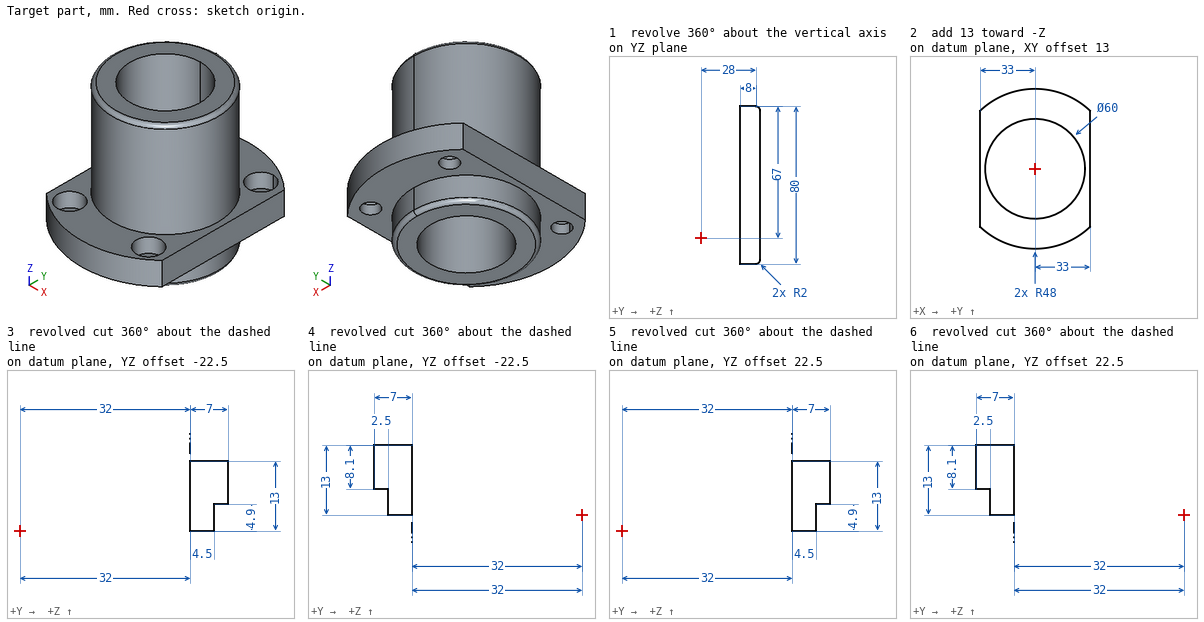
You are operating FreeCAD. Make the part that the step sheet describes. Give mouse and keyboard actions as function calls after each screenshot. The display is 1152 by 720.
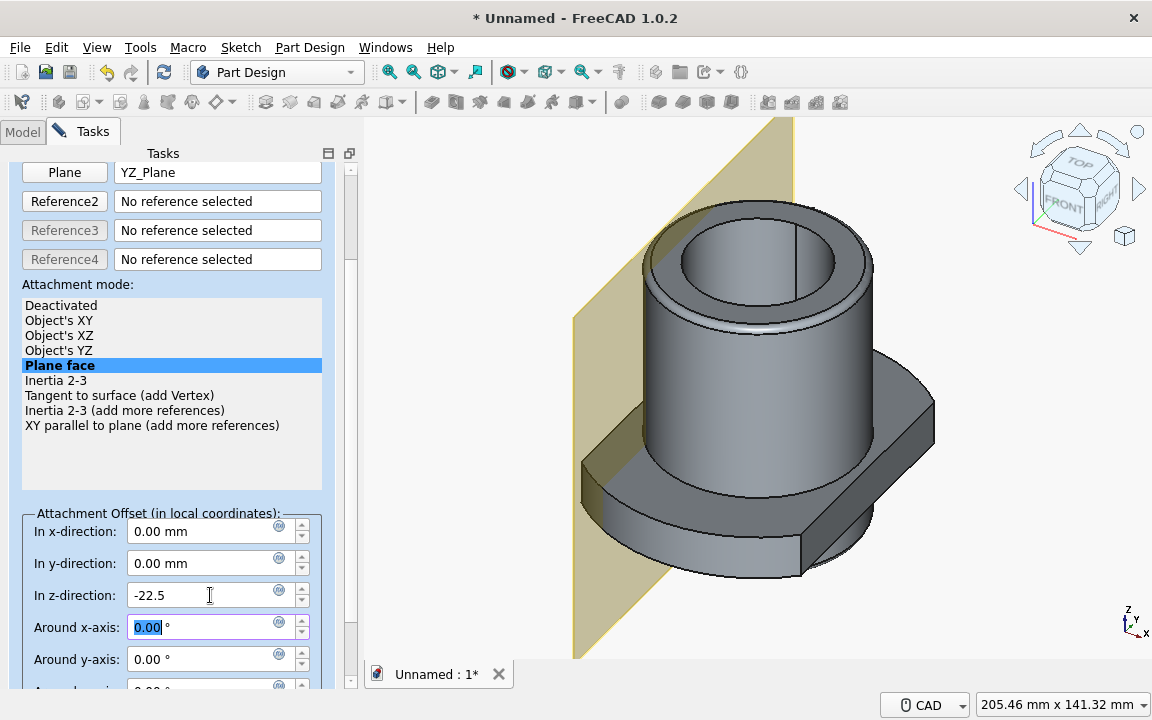
scroll(351, 426, up, 3)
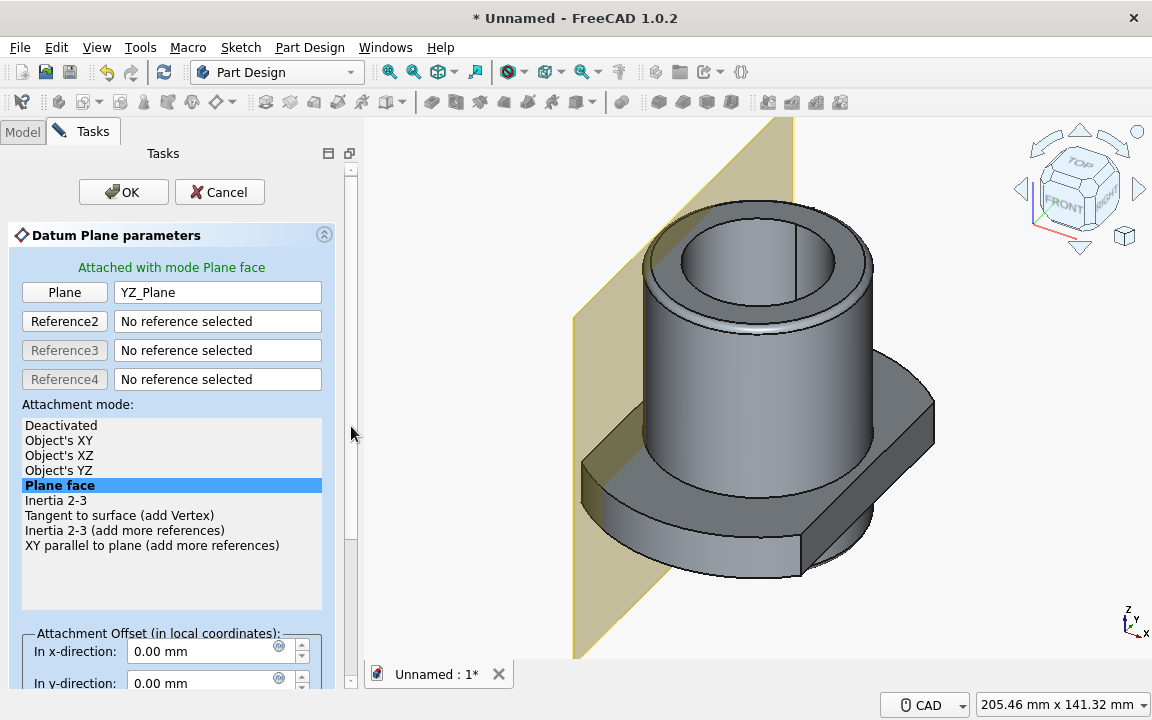
click(124, 192)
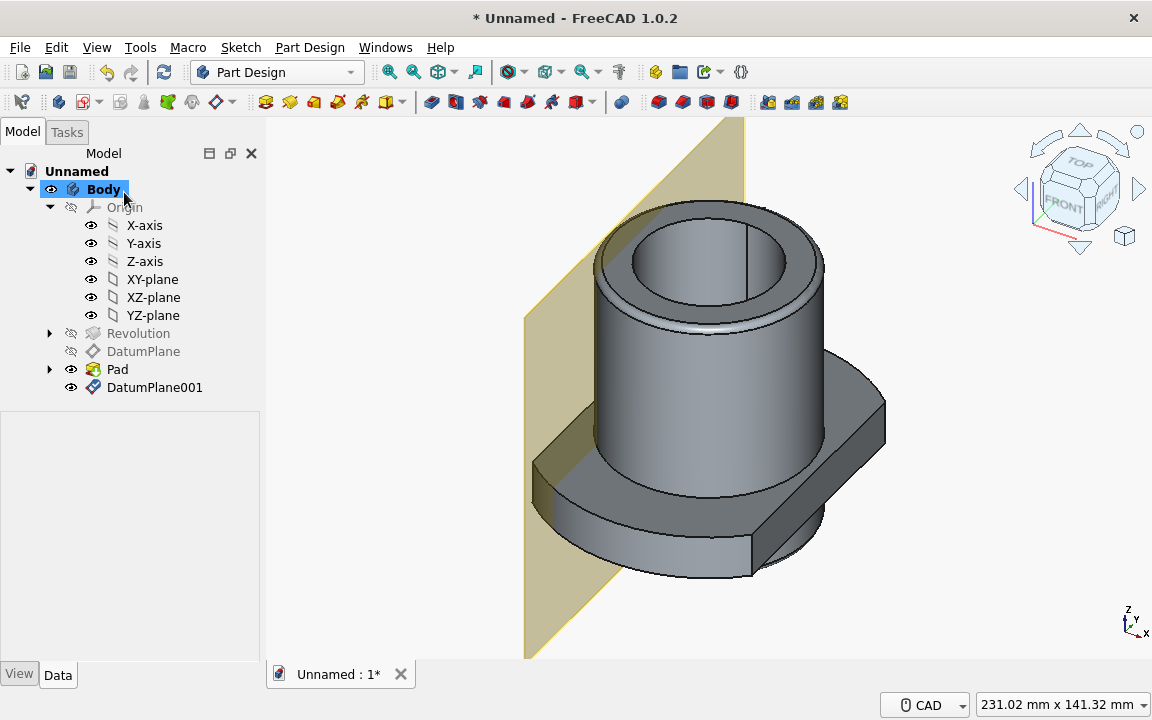
click(116, 387)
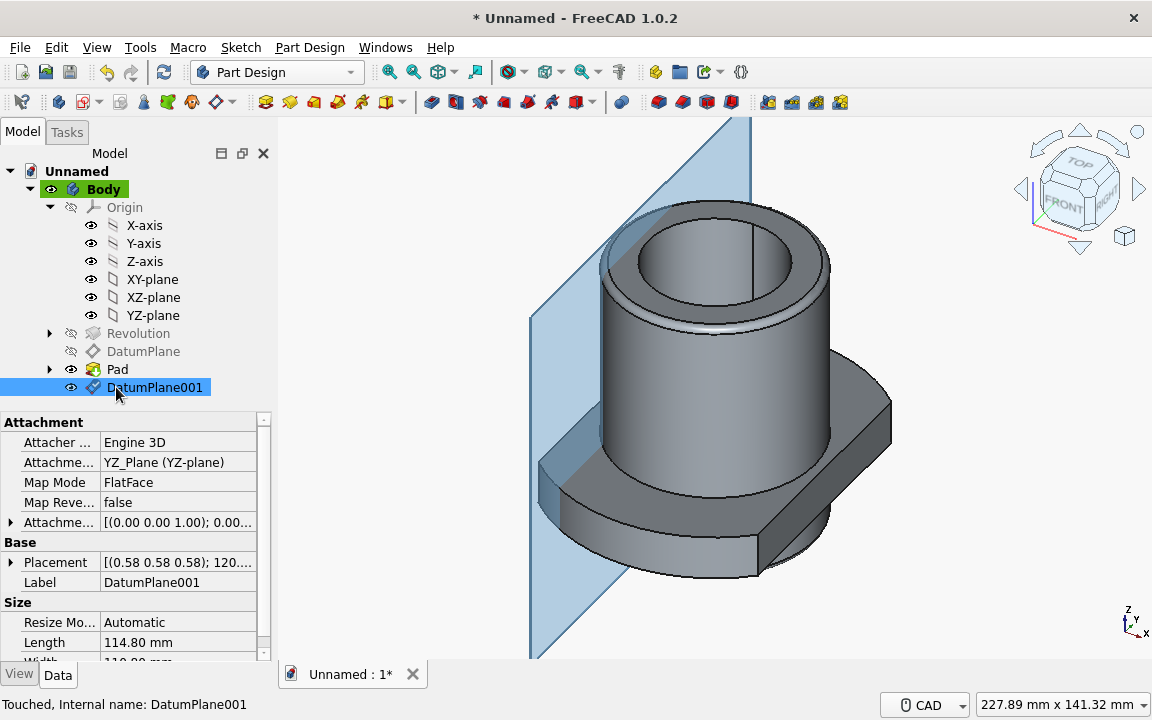
click(84, 102)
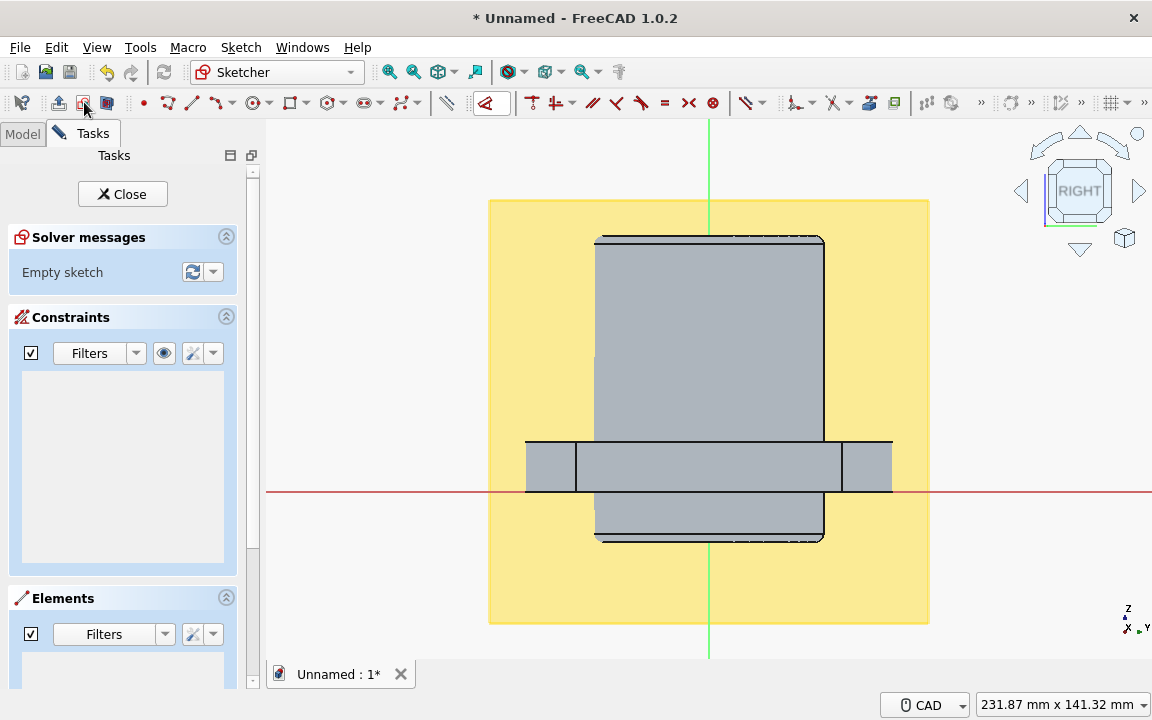
click(108, 104)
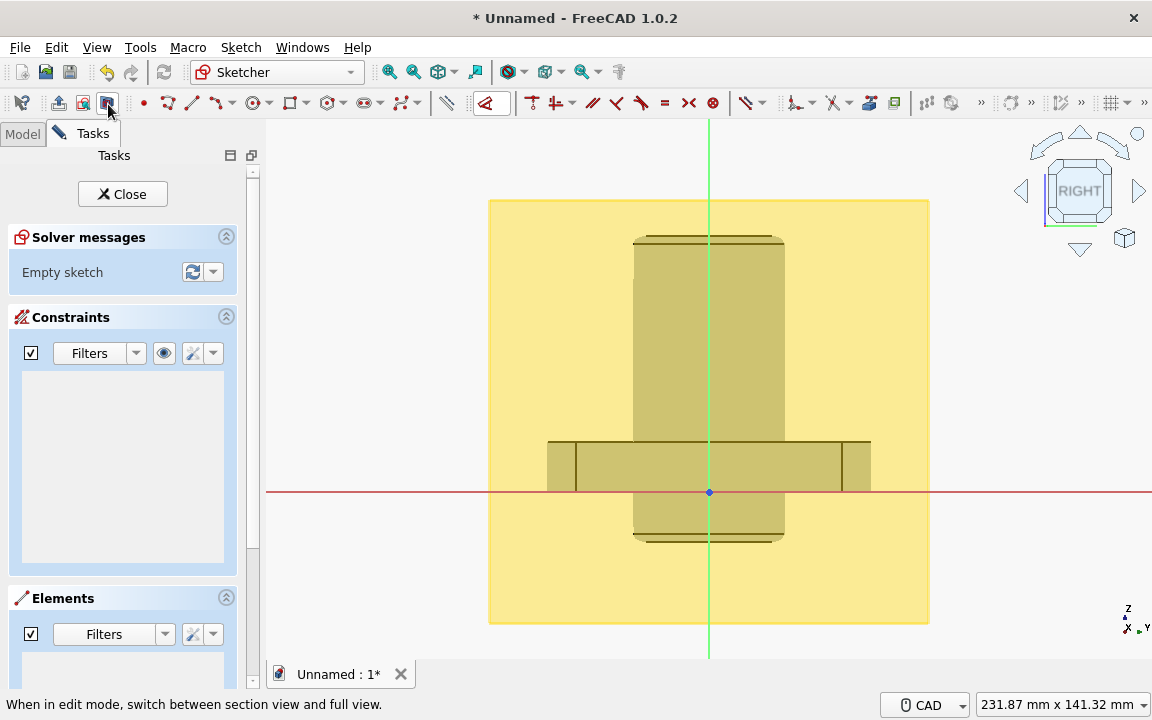
scroll(845, 487, up, 6)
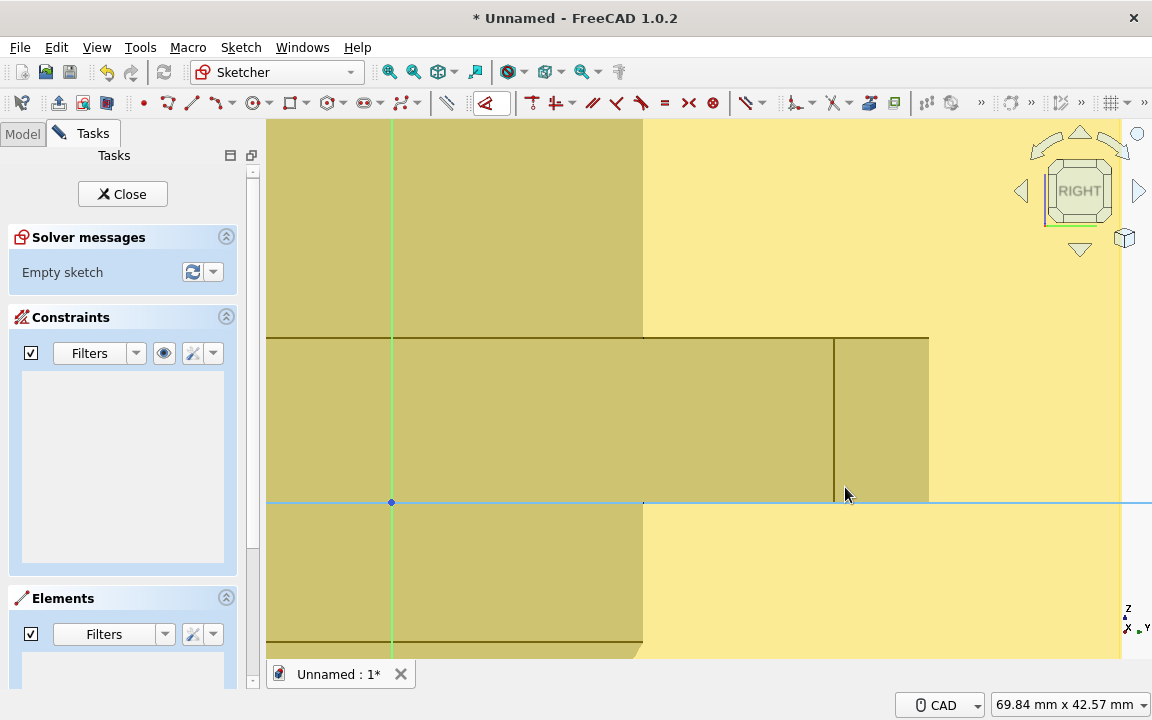
click(168, 104)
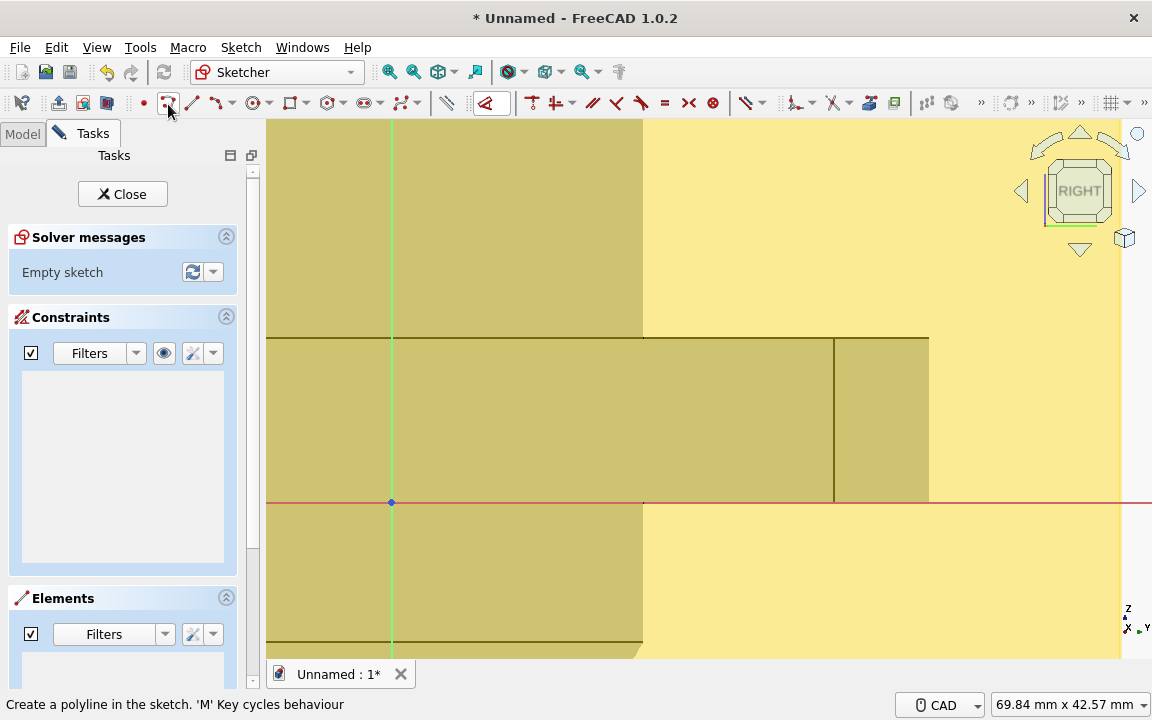
click(798, 503)
click(855, 494)
click(855, 440)
click(887, 440)
click(887, 338)
click(798, 338)
click(798, 503)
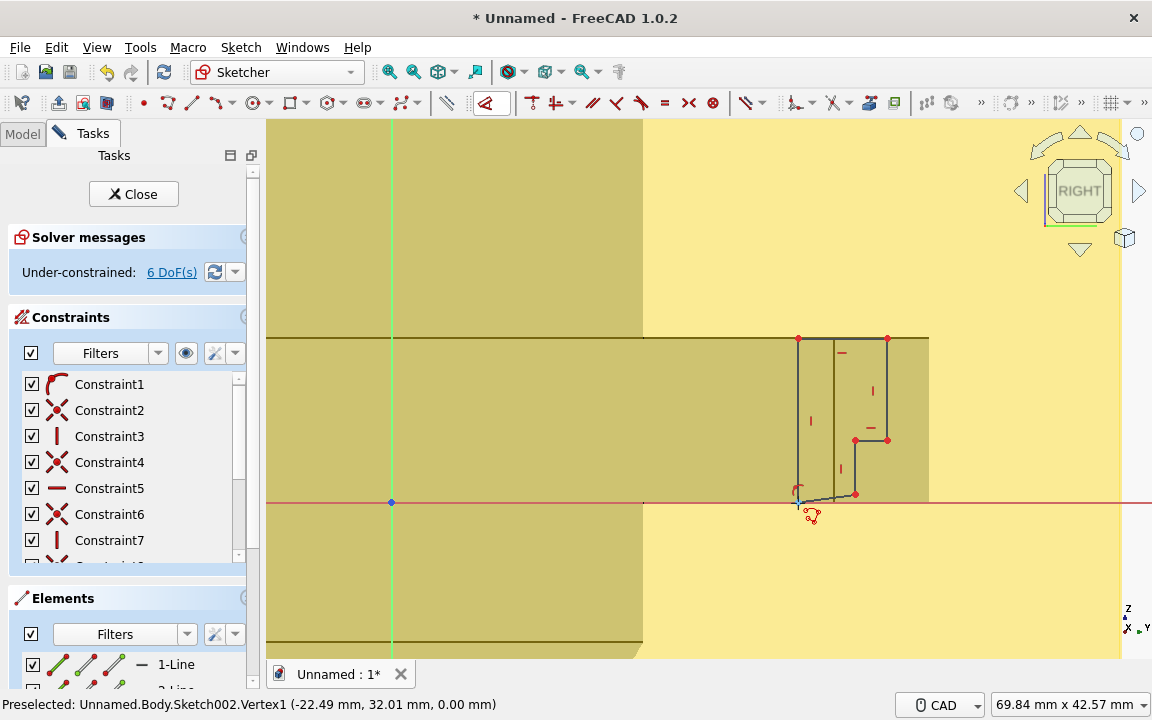
click(192, 104)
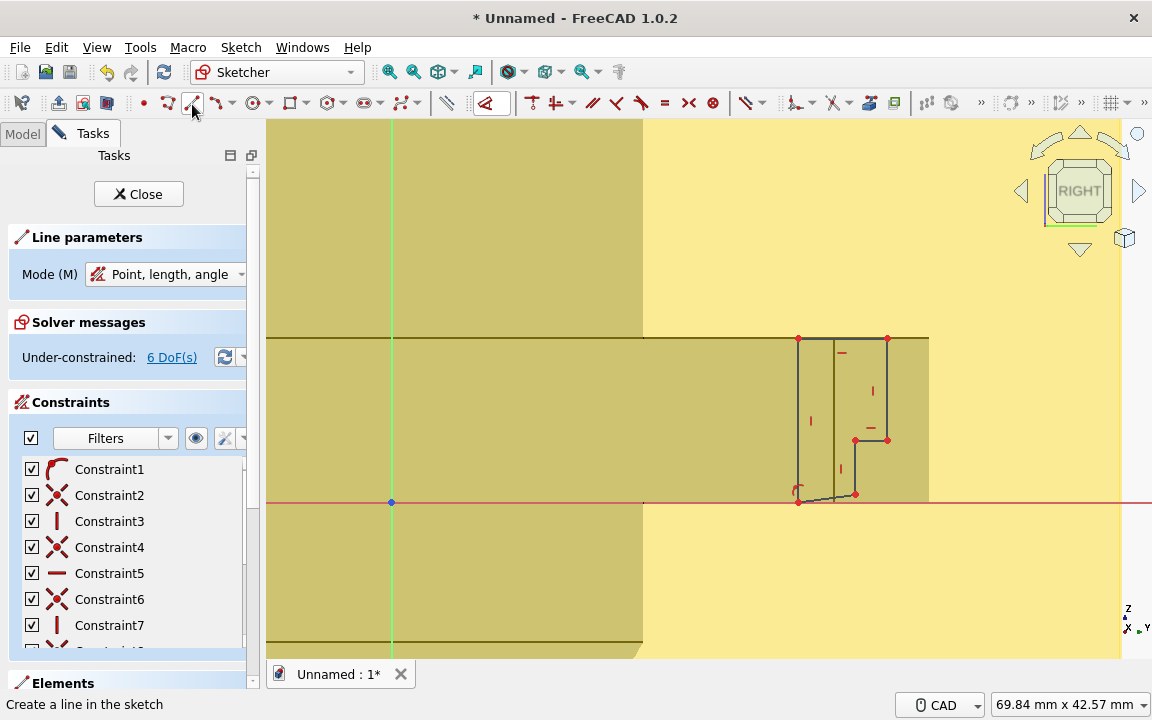
click(798, 321)
click(798, 272)
key(Escape)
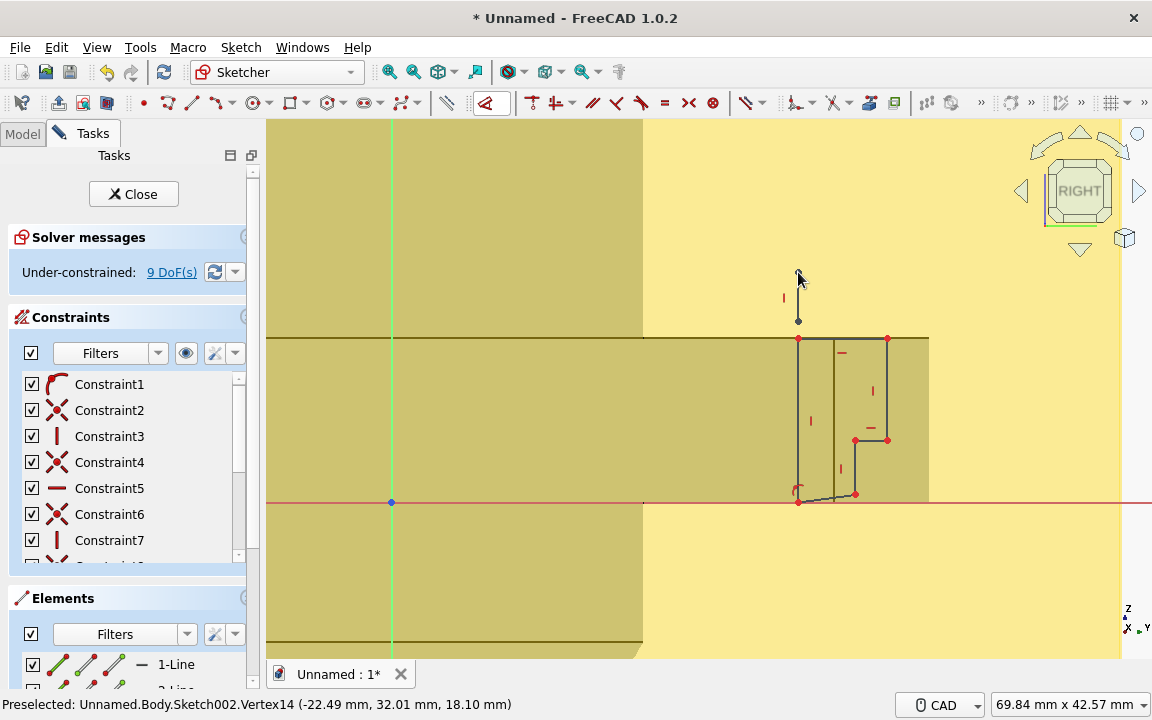
click(798, 307)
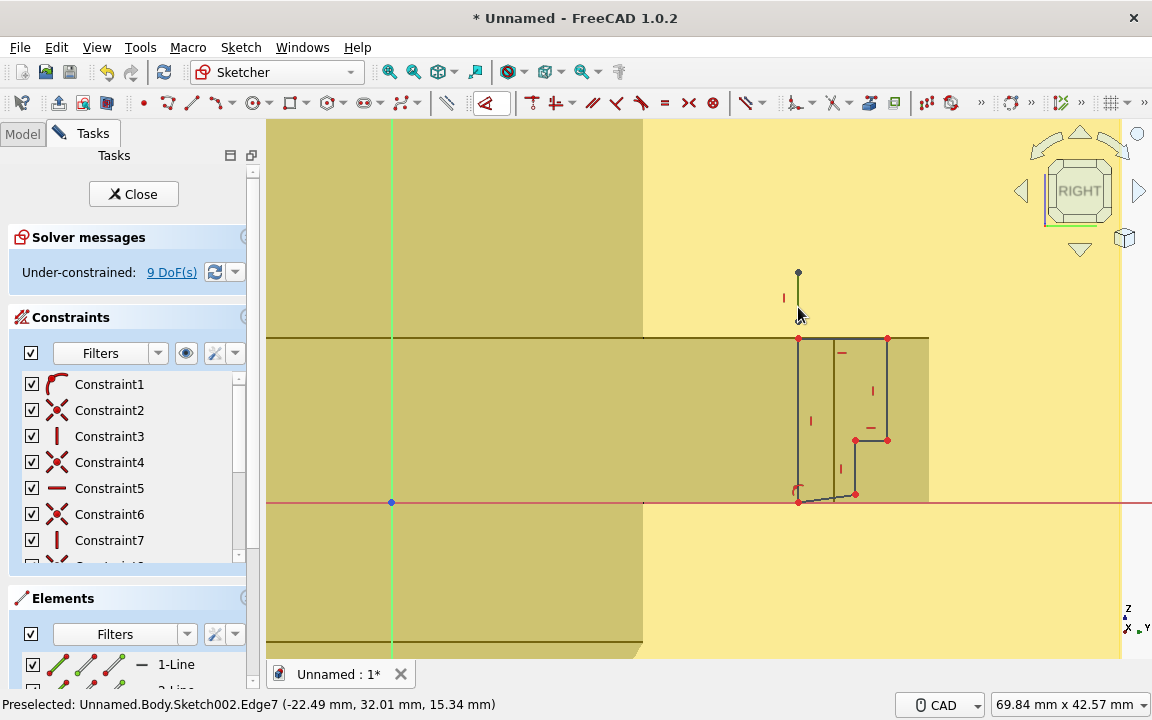
click(448, 104)